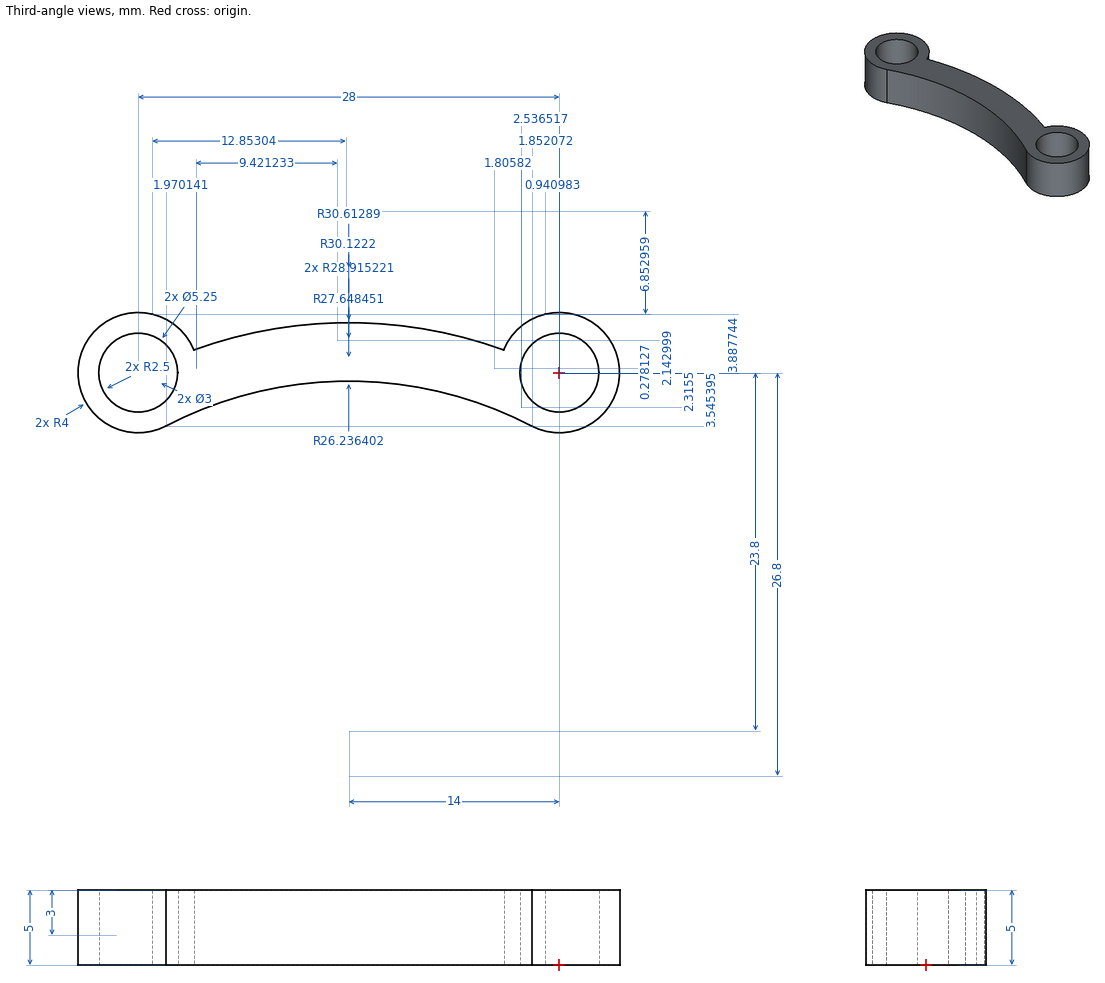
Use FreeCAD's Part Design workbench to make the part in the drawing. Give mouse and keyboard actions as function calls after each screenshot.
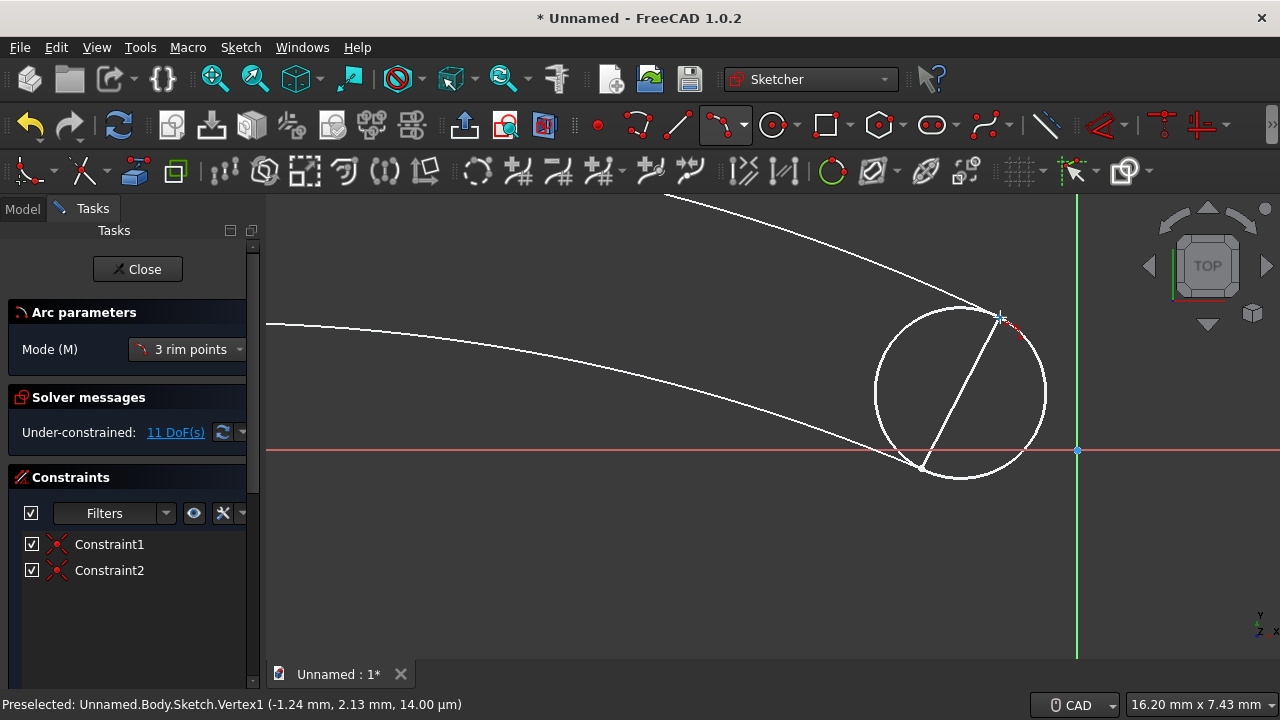
scroll(922, 470, down, 6)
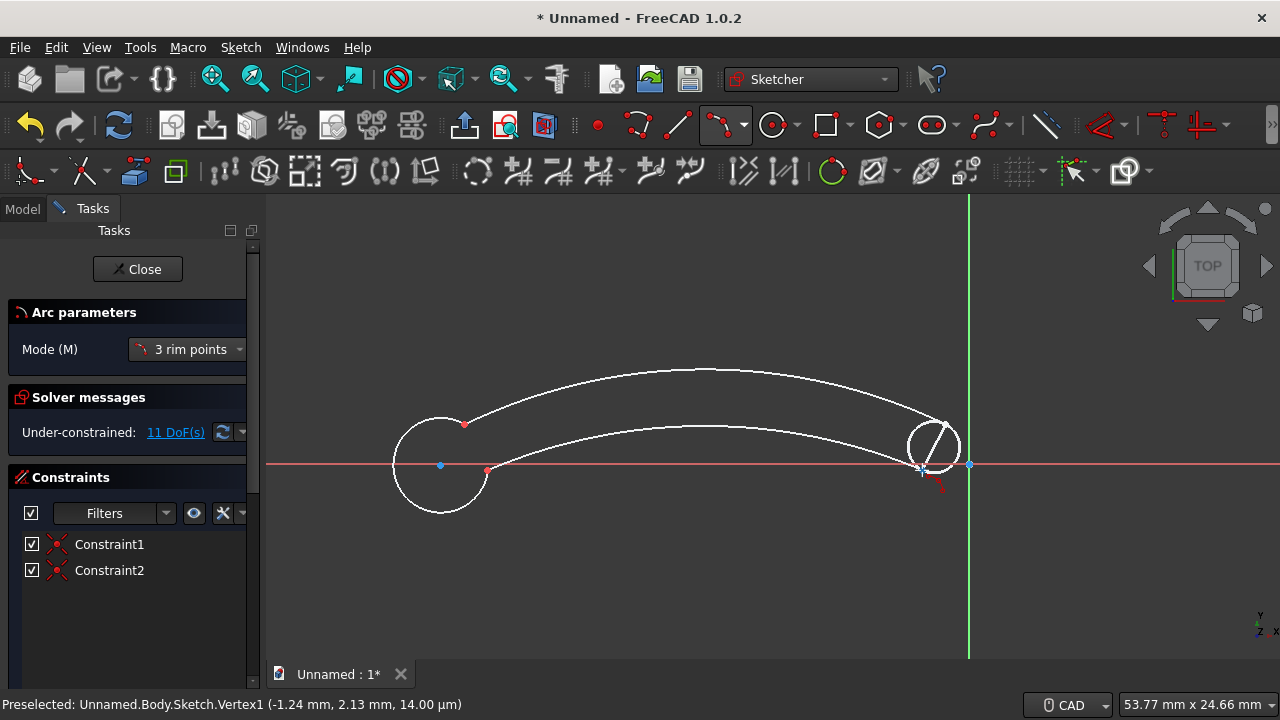
click(1011, 486)
key(Escape)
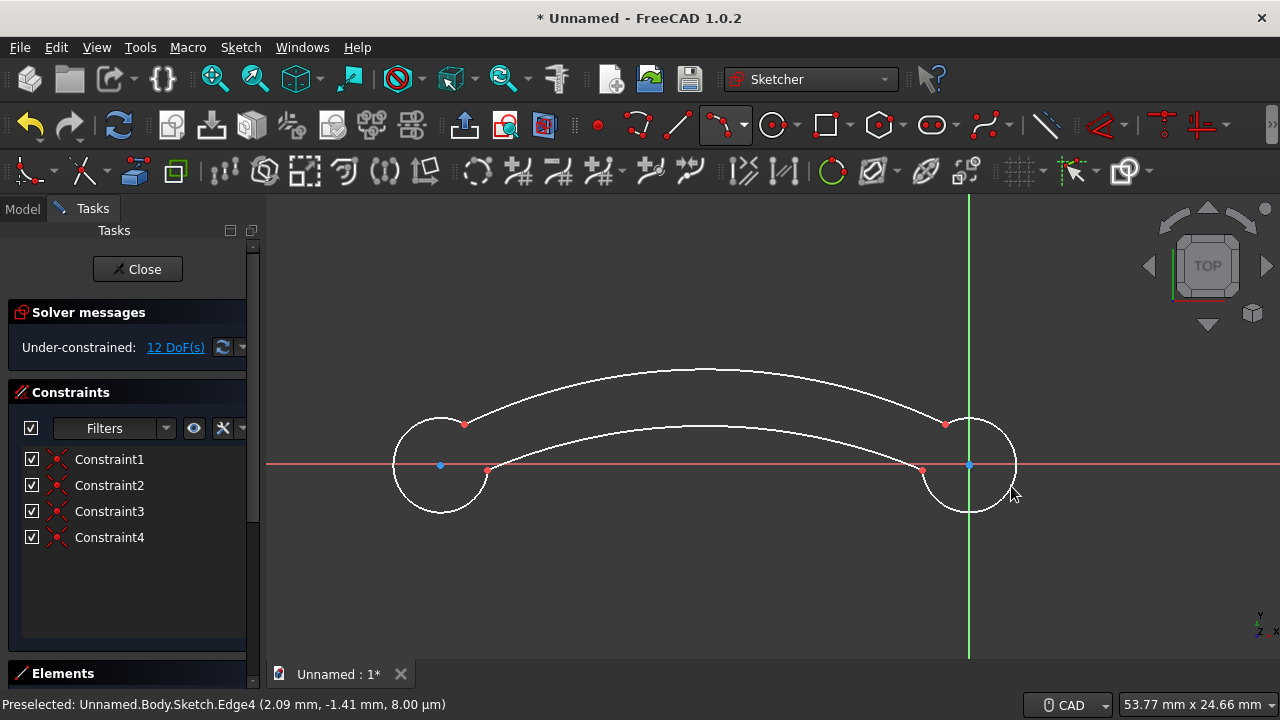
drag(959, 454, 979, 475)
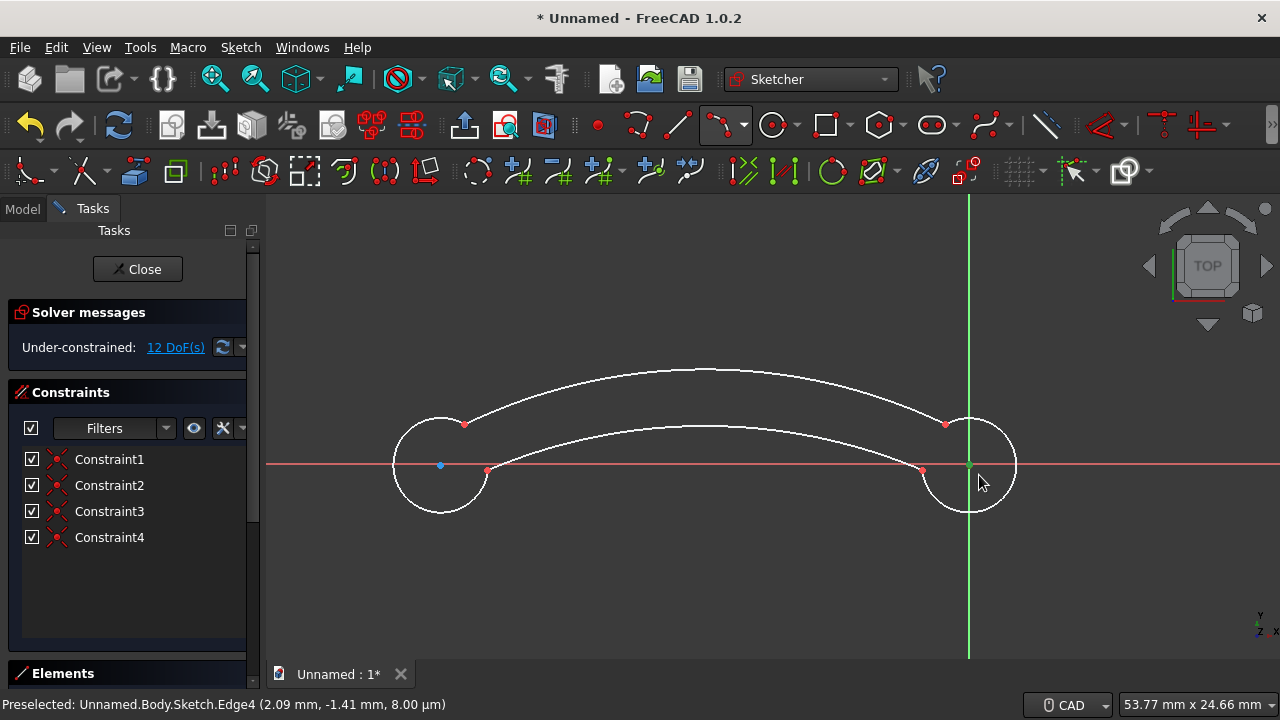
click(1162, 126)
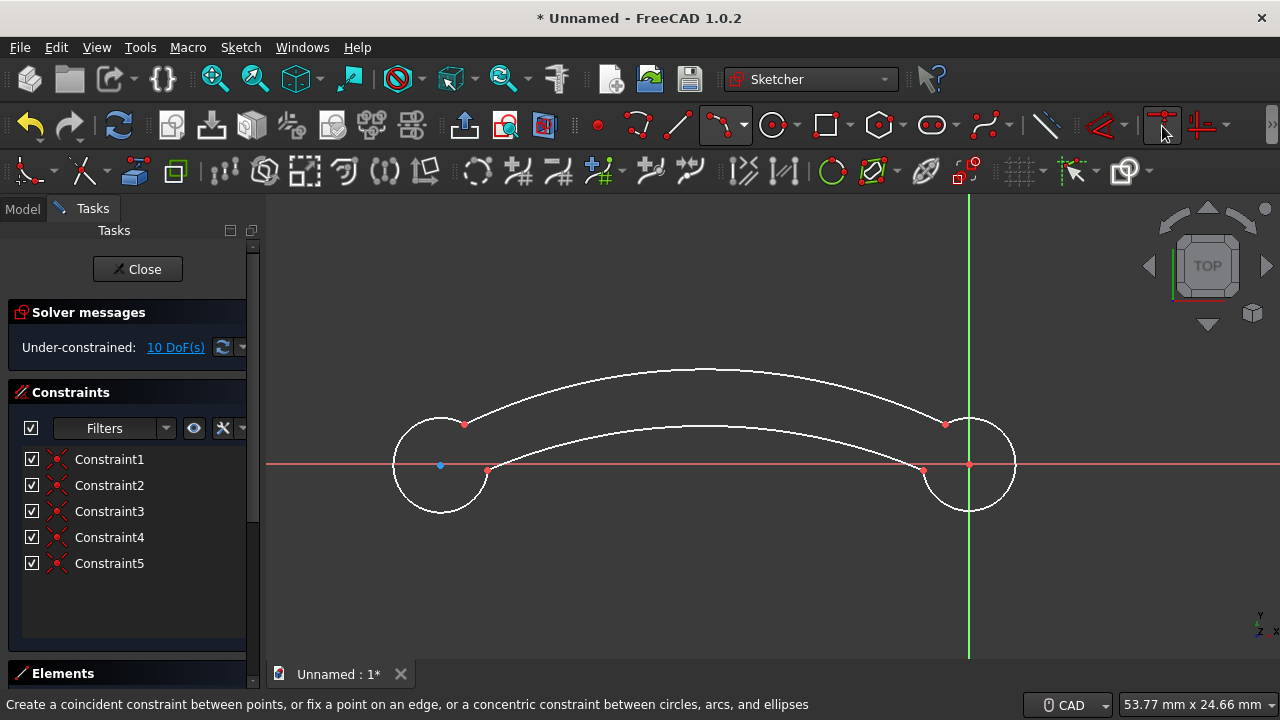
click(804, 378)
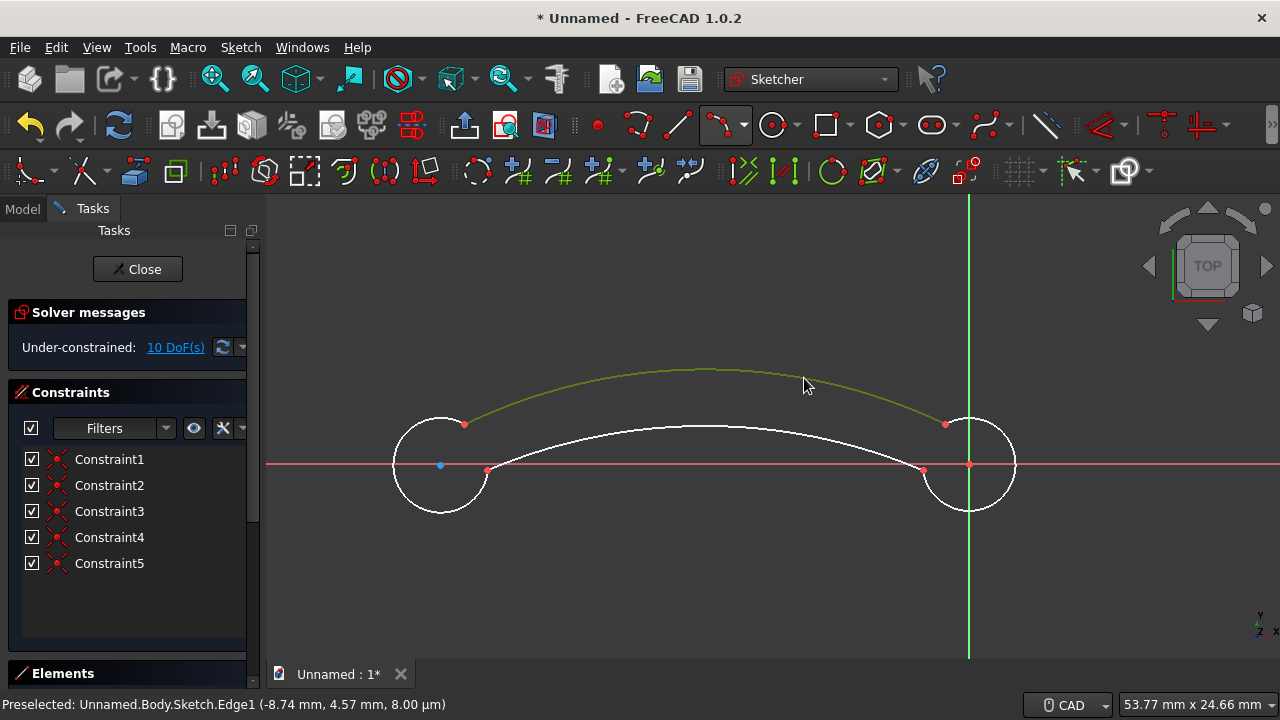
click(795, 433)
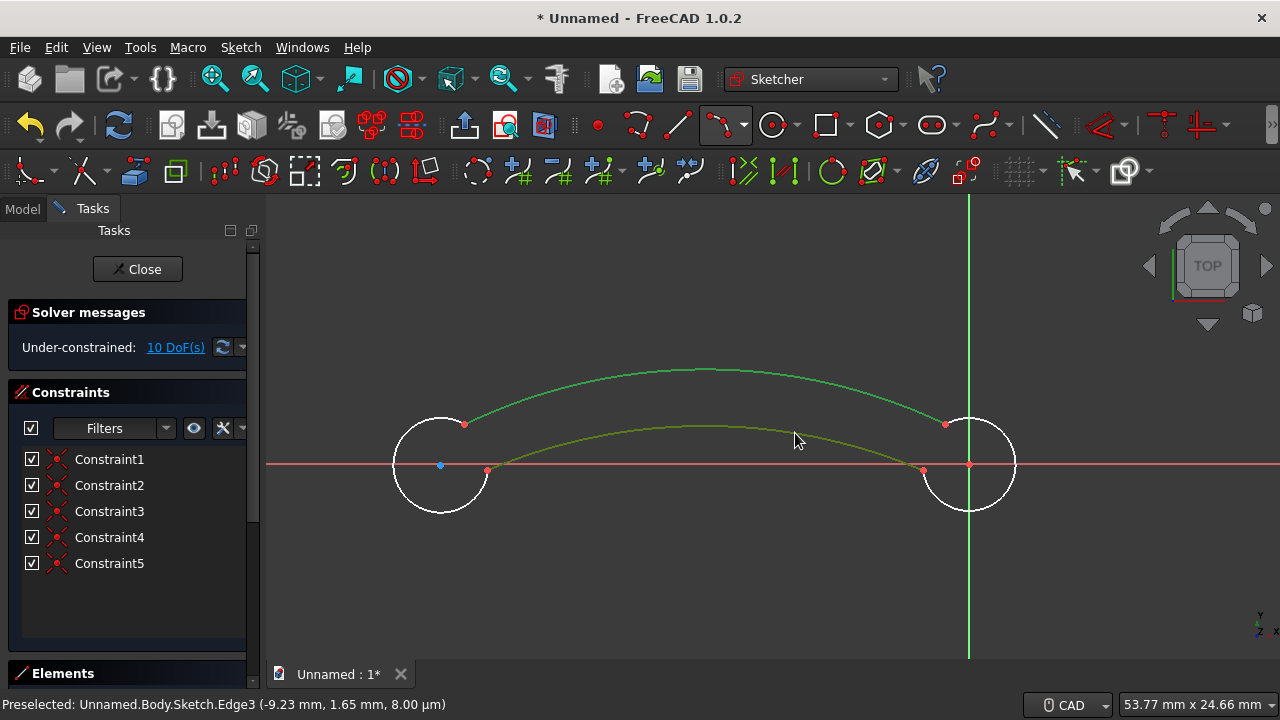
key(e)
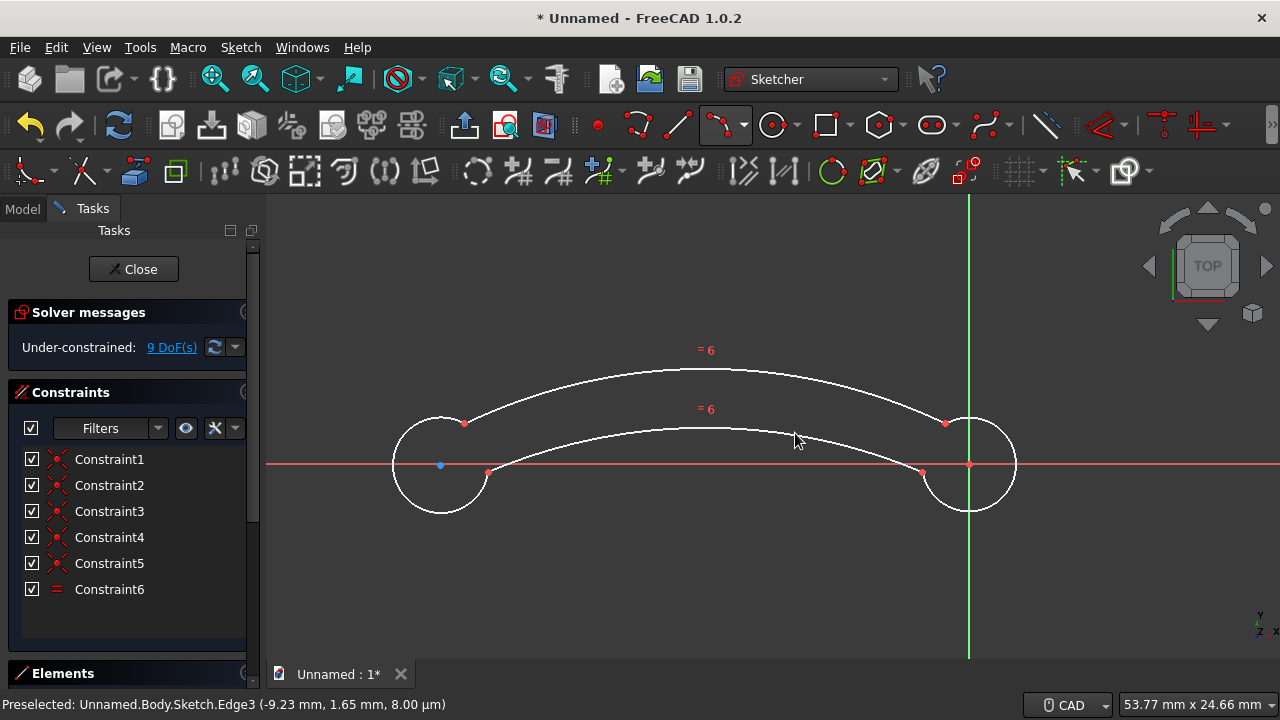
click(401, 439)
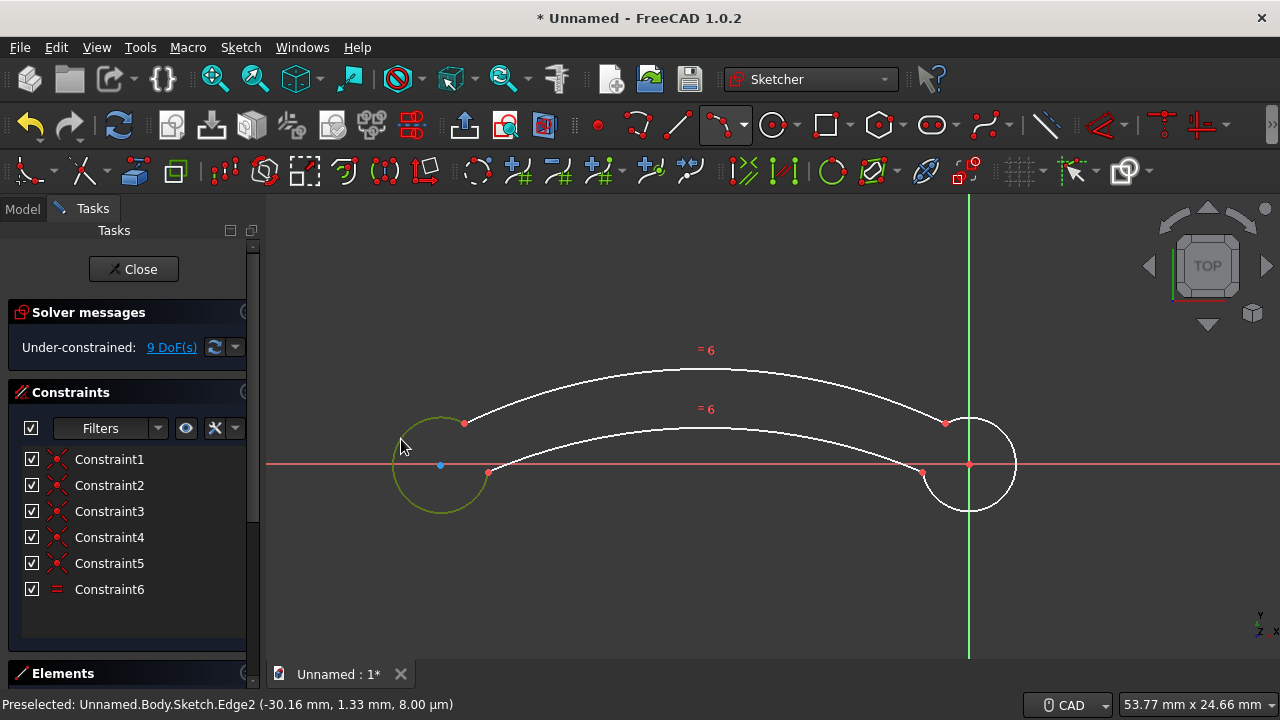
click(1009, 439)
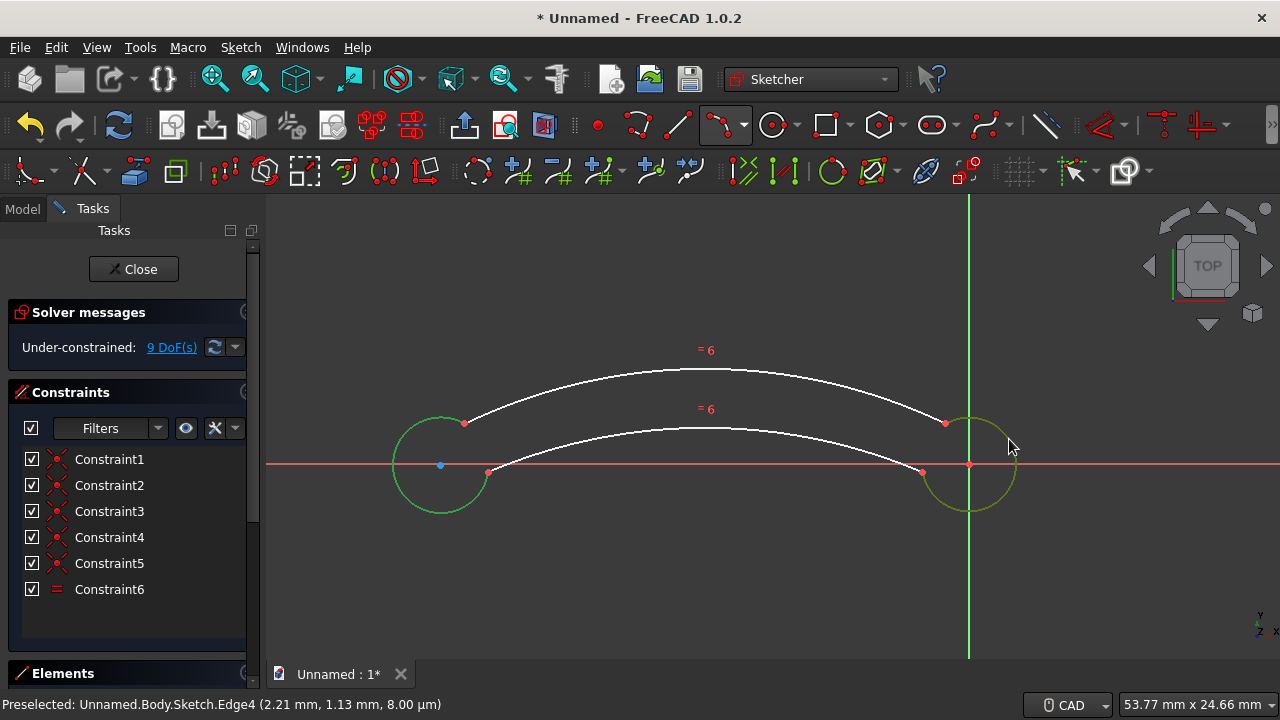
key(e)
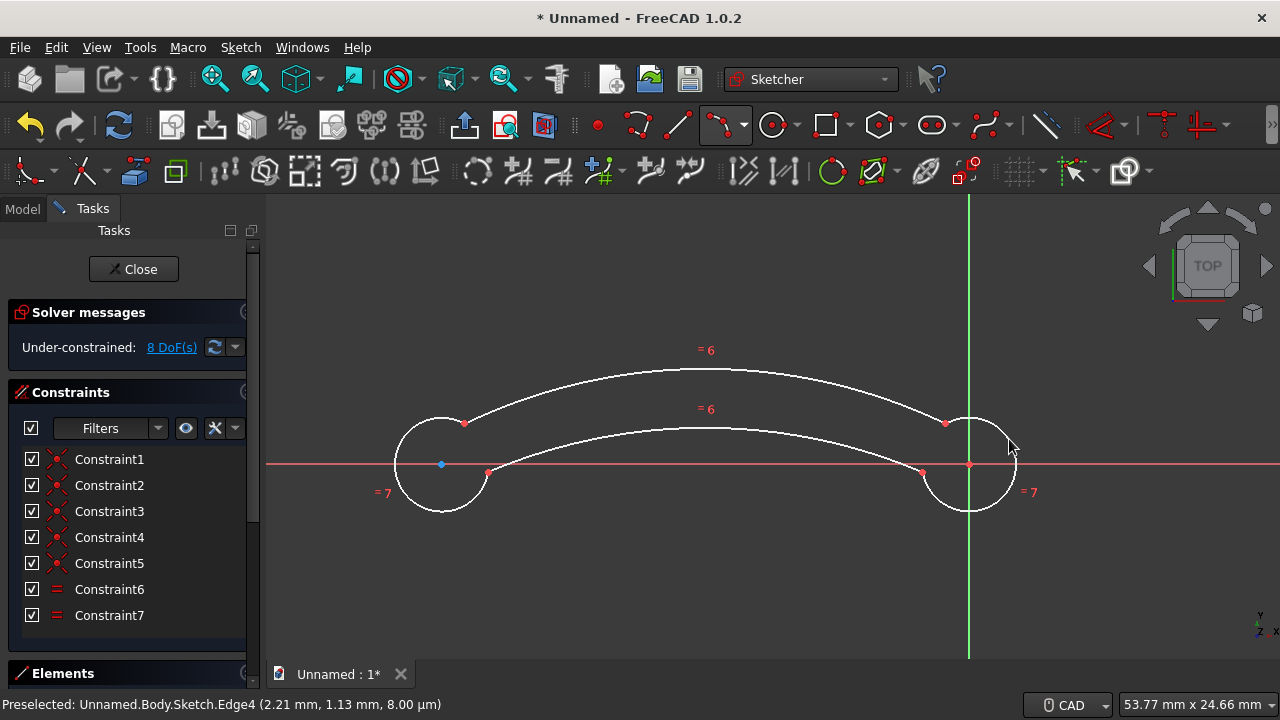
click(442, 465)